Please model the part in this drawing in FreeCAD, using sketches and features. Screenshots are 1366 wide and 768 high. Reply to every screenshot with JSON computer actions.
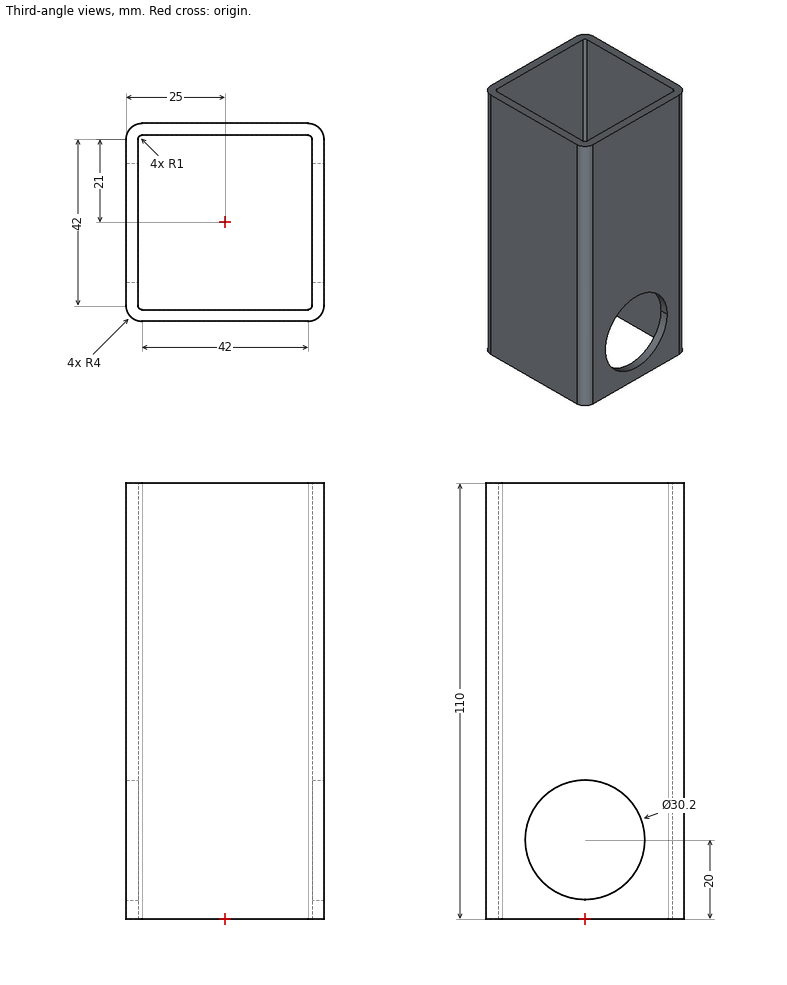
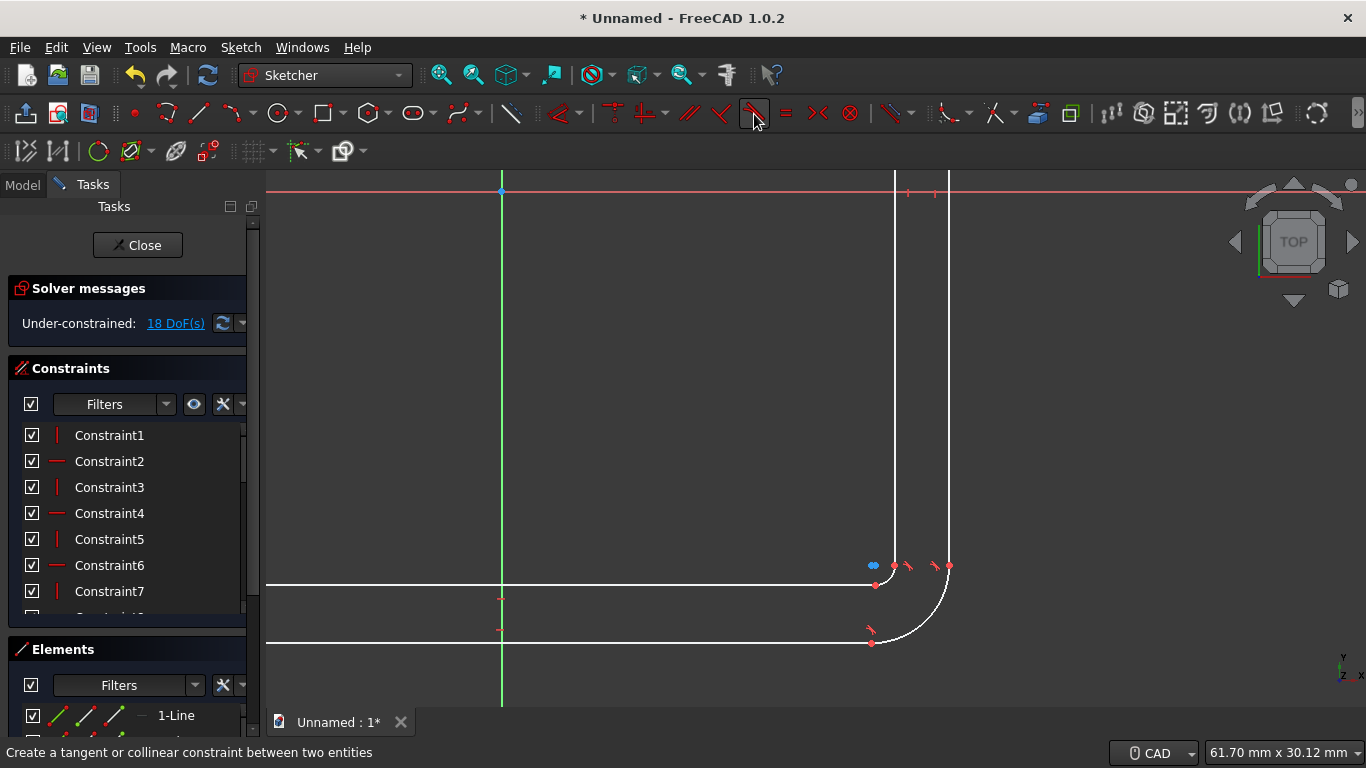
{"action": "left_click", "coordinate": [651, 585]}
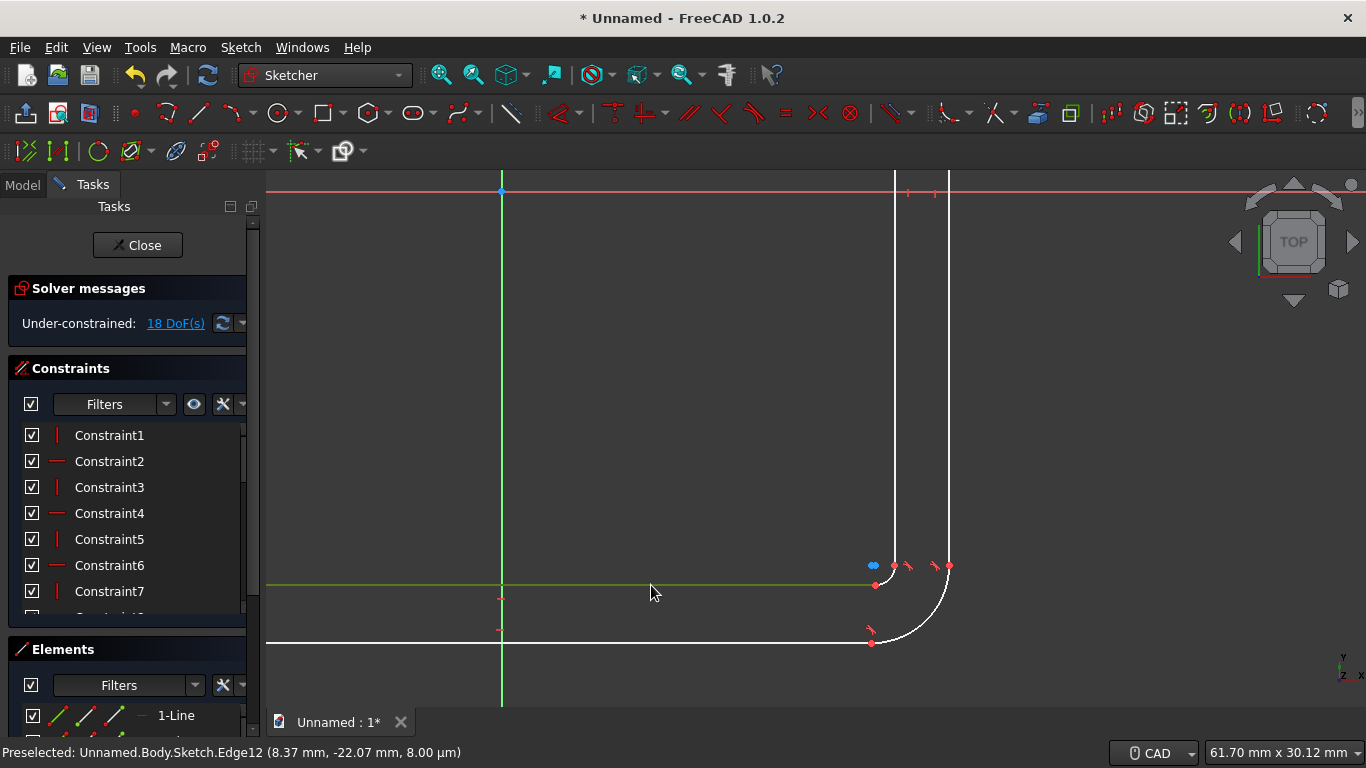
{"action": "scroll", "coordinate": [885, 583], "scroll_direction": "up", "scroll_amount": 3}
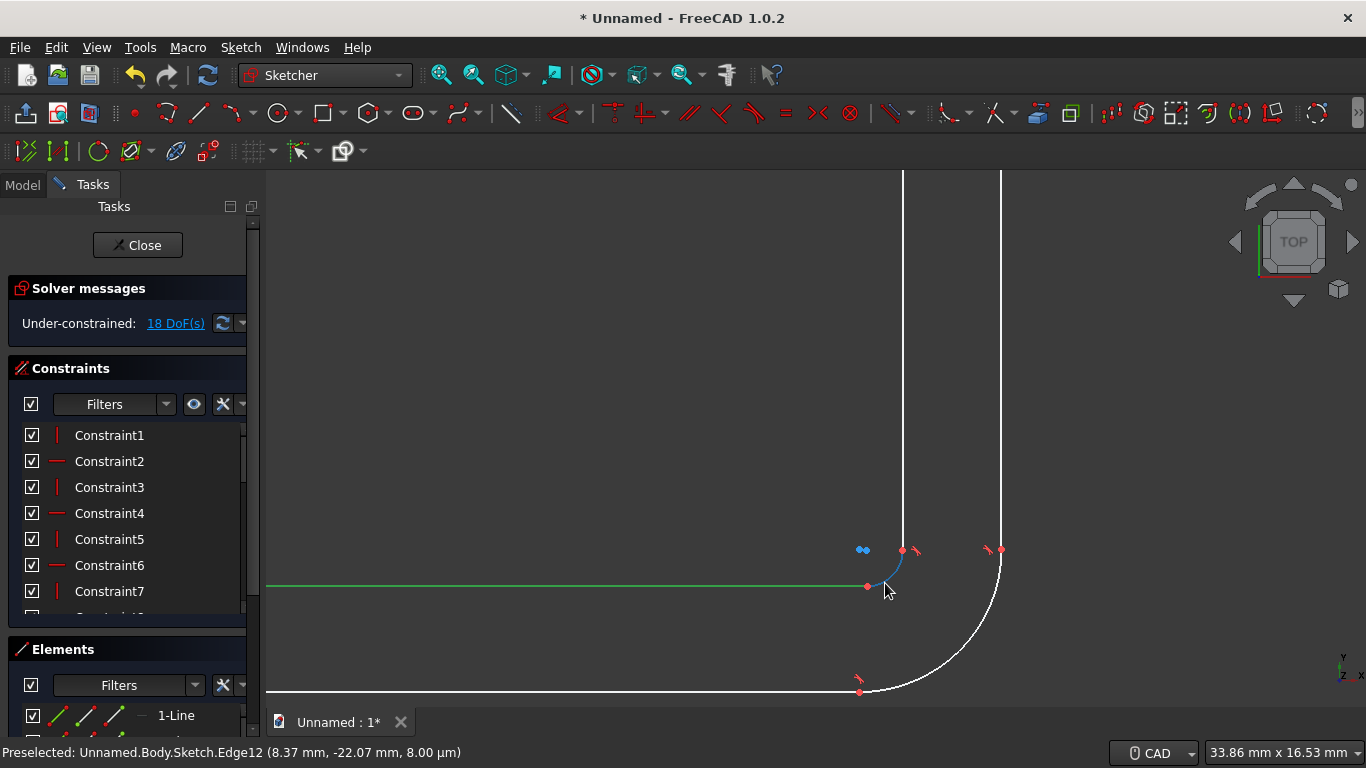
{"action": "left_click", "coordinate": [884, 582]}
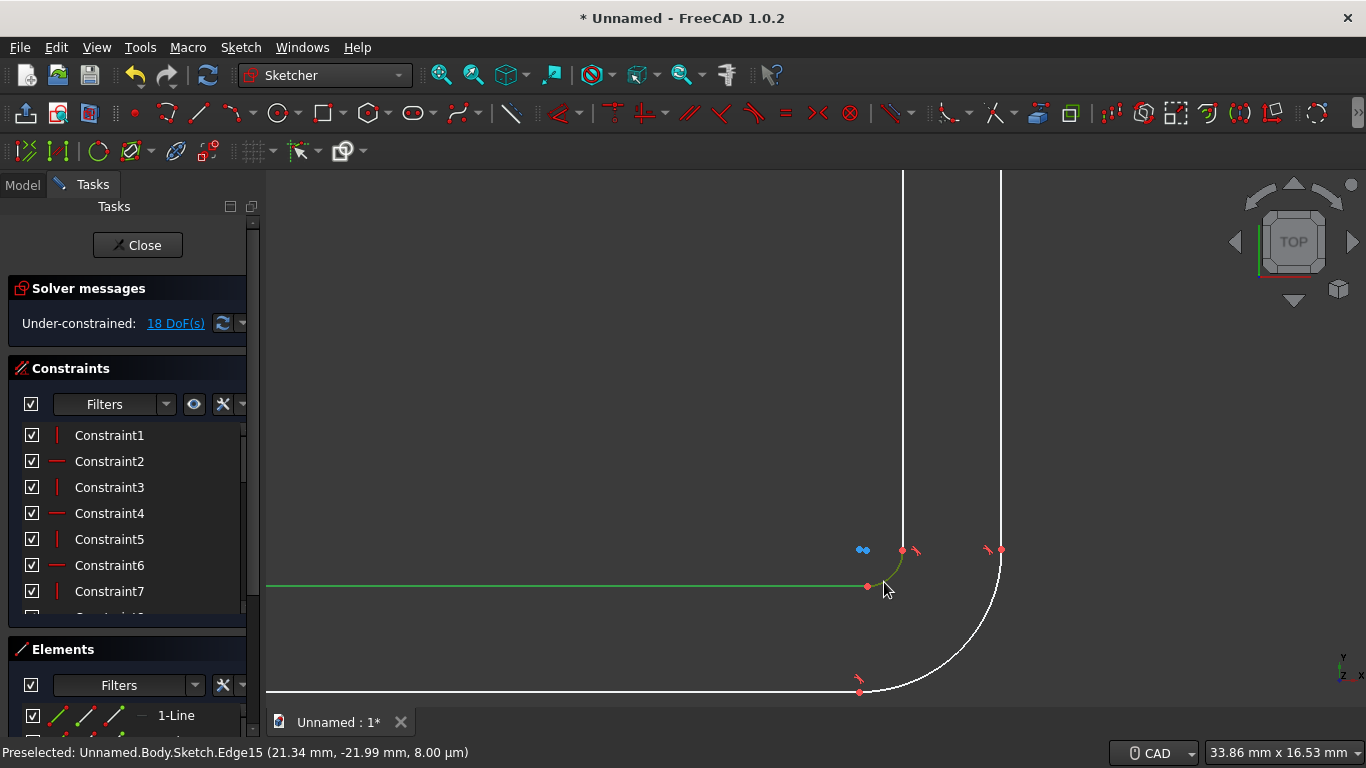
{"action": "left_click", "coordinate": [754, 114]}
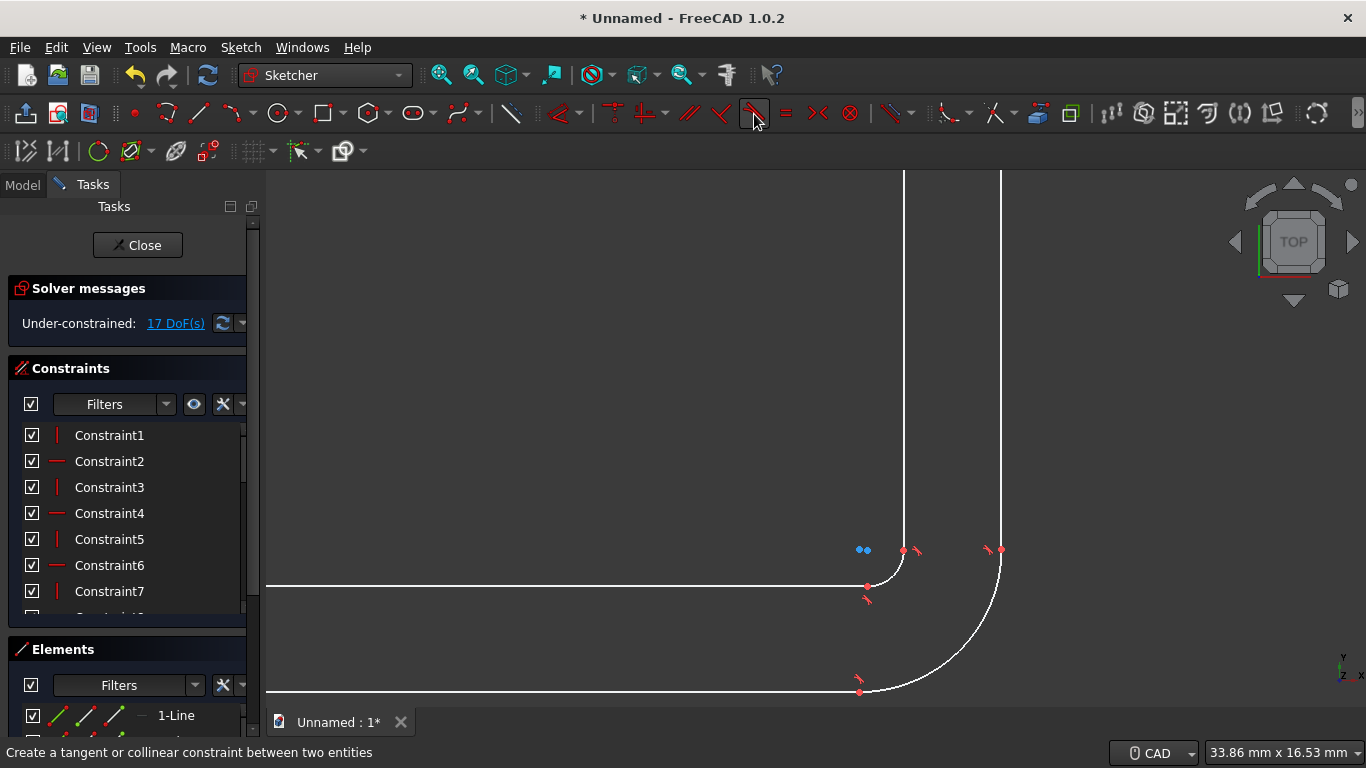
{"action": "scroll", "coordinate": [889, 582], "scroll_direction": "down", "scroll_amount": 8}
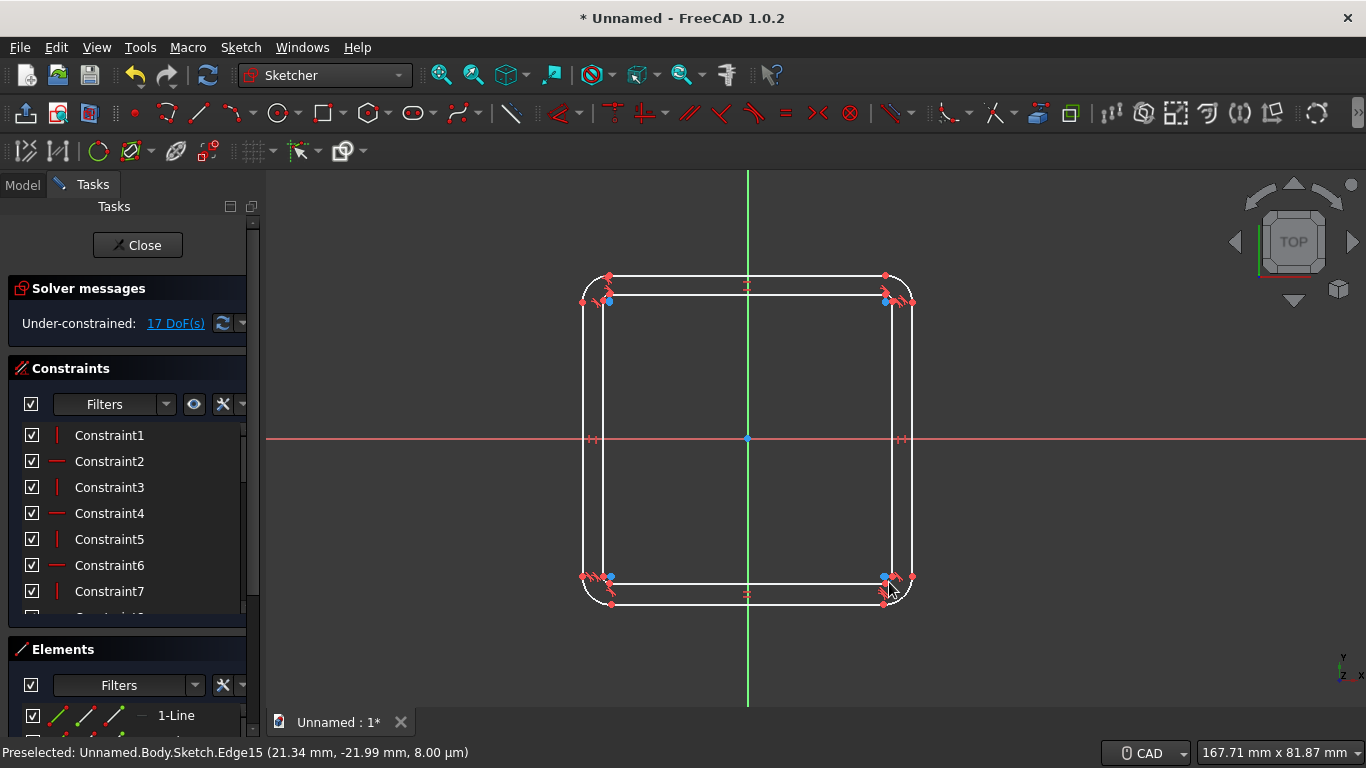
{"action": "left_click", "coordinate": [803, 583]}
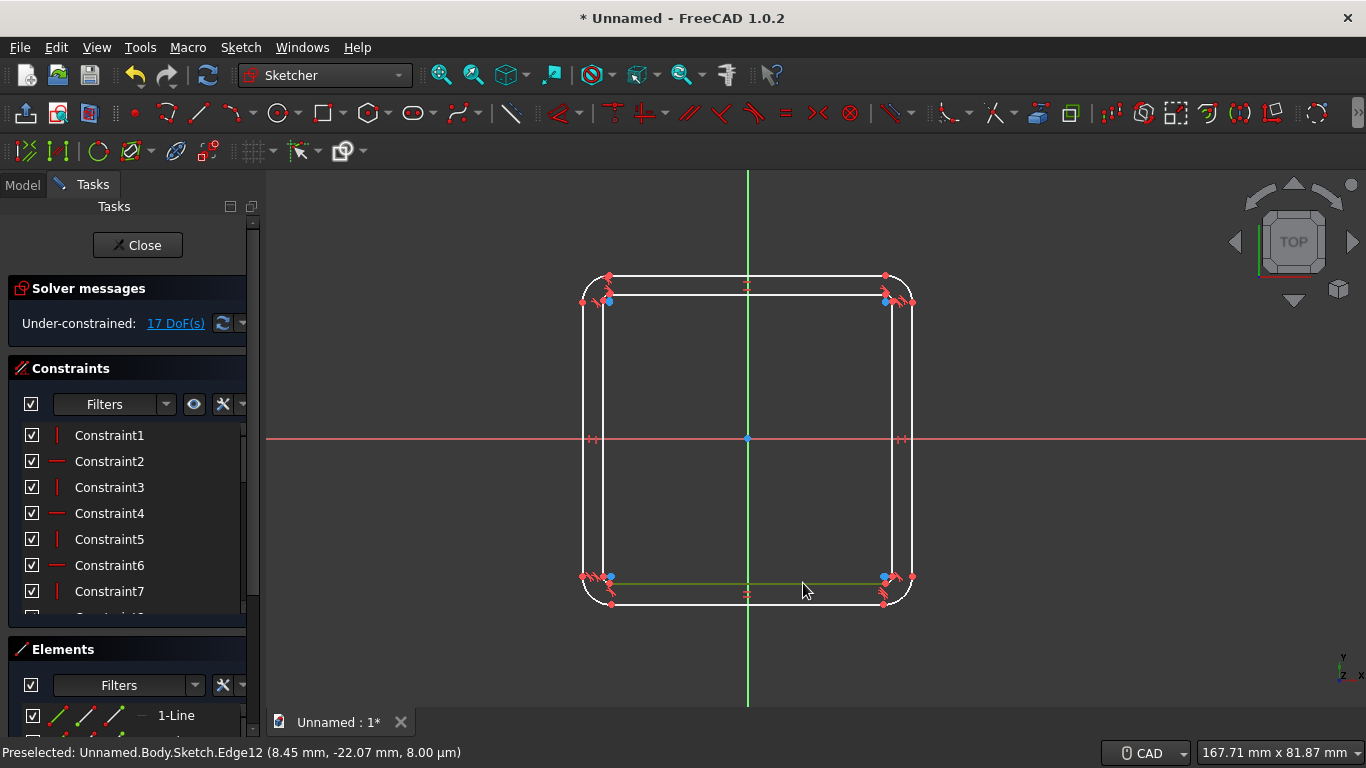
{"action": "scroll", "coordinate": [605, 581], "scroll_direction": "up", "scroll_amount": 5}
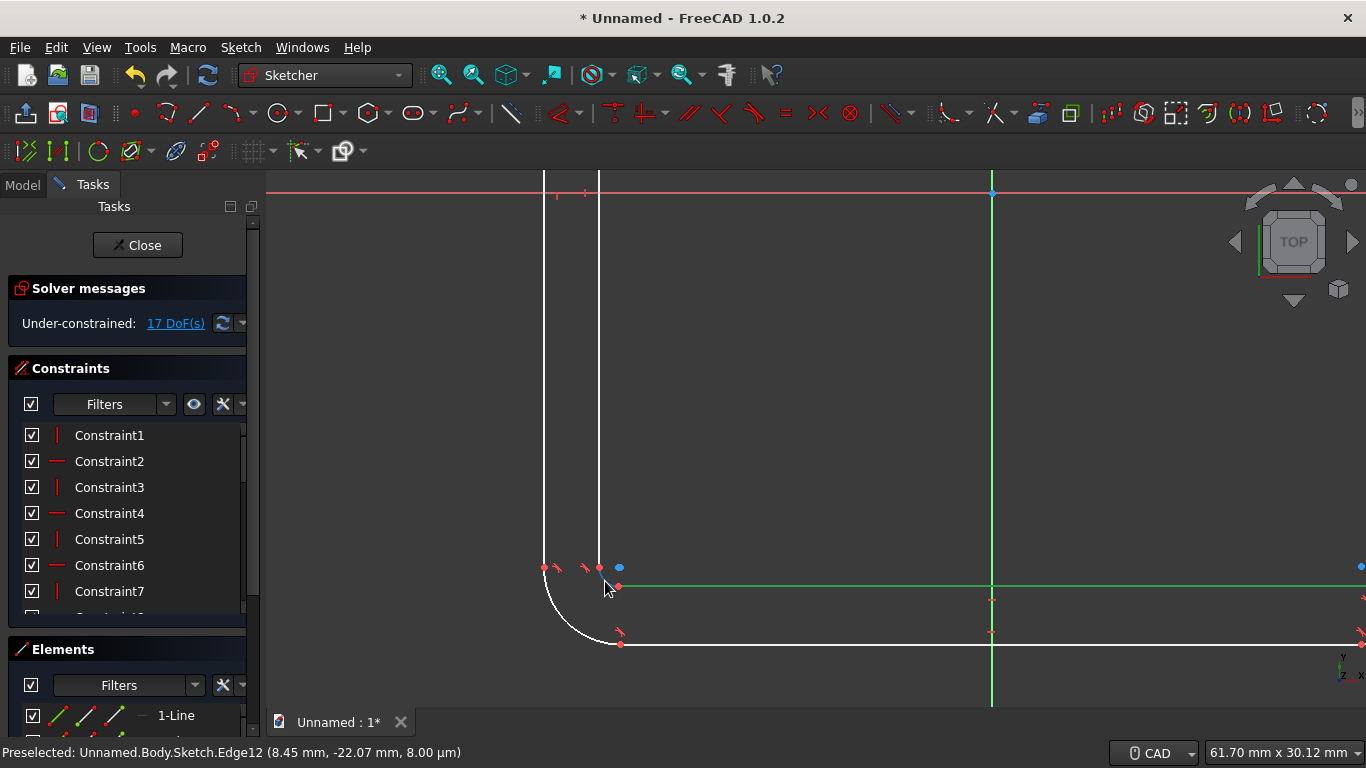
{"action": "left_click", "coordinate": [605, 581]}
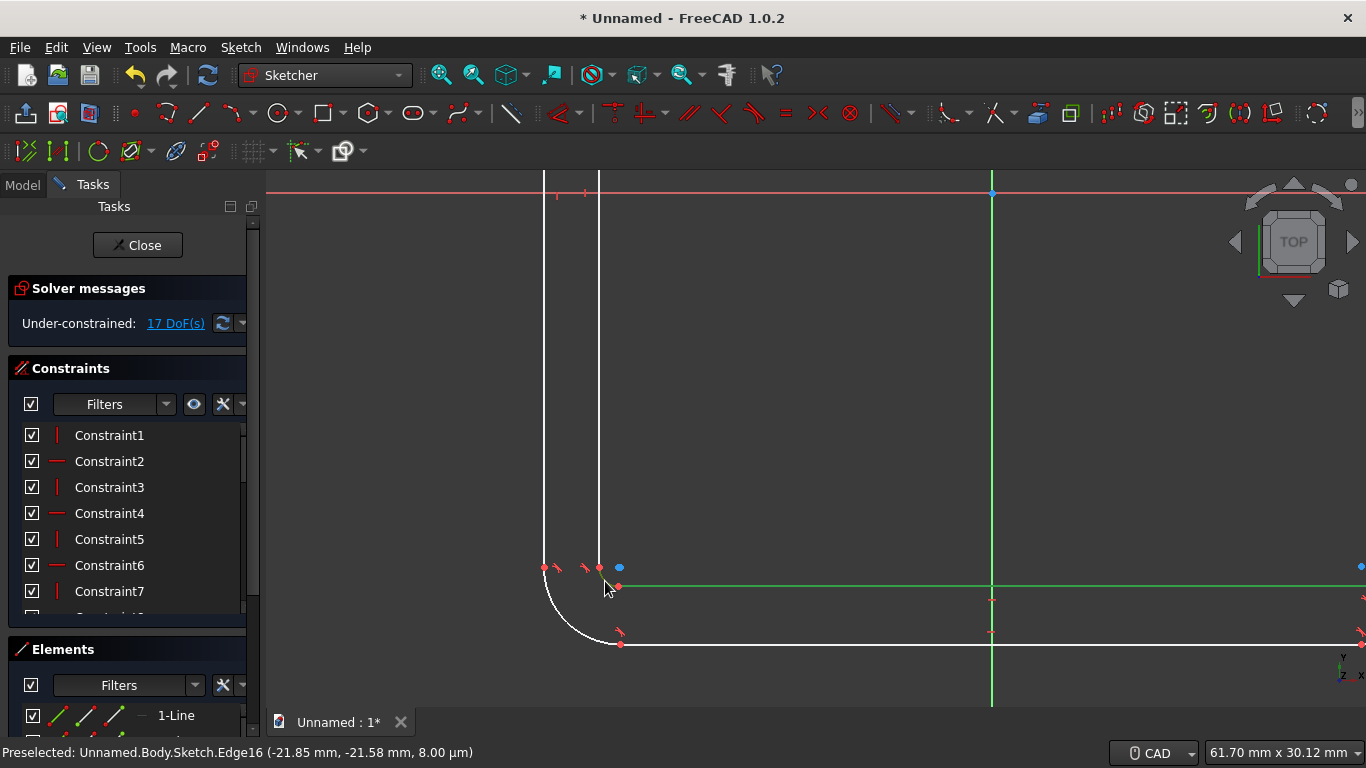
{"action": "left_click", "coordinate": [754, 114]}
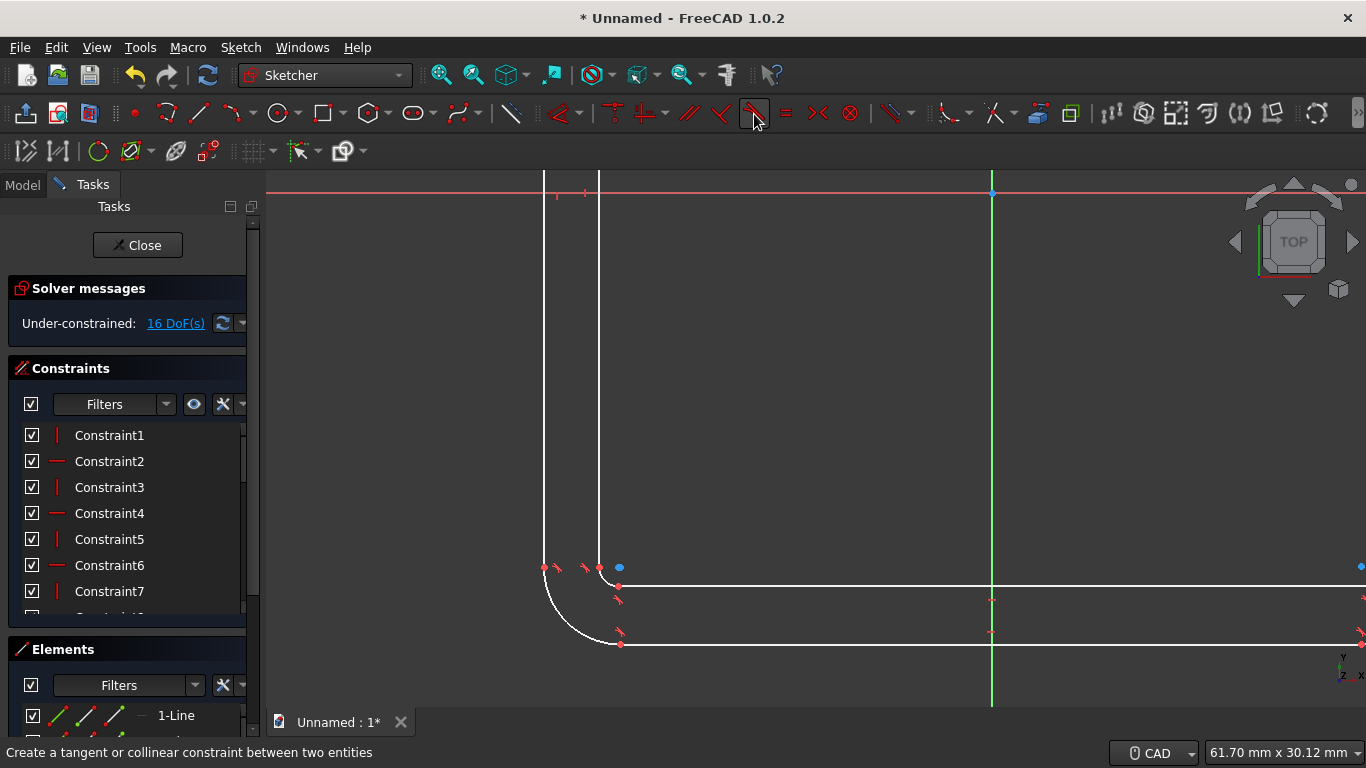
{"action": "scroll", "coordinate": [605, 581], "scroll_direction": "down", "scroll_amount": 5}